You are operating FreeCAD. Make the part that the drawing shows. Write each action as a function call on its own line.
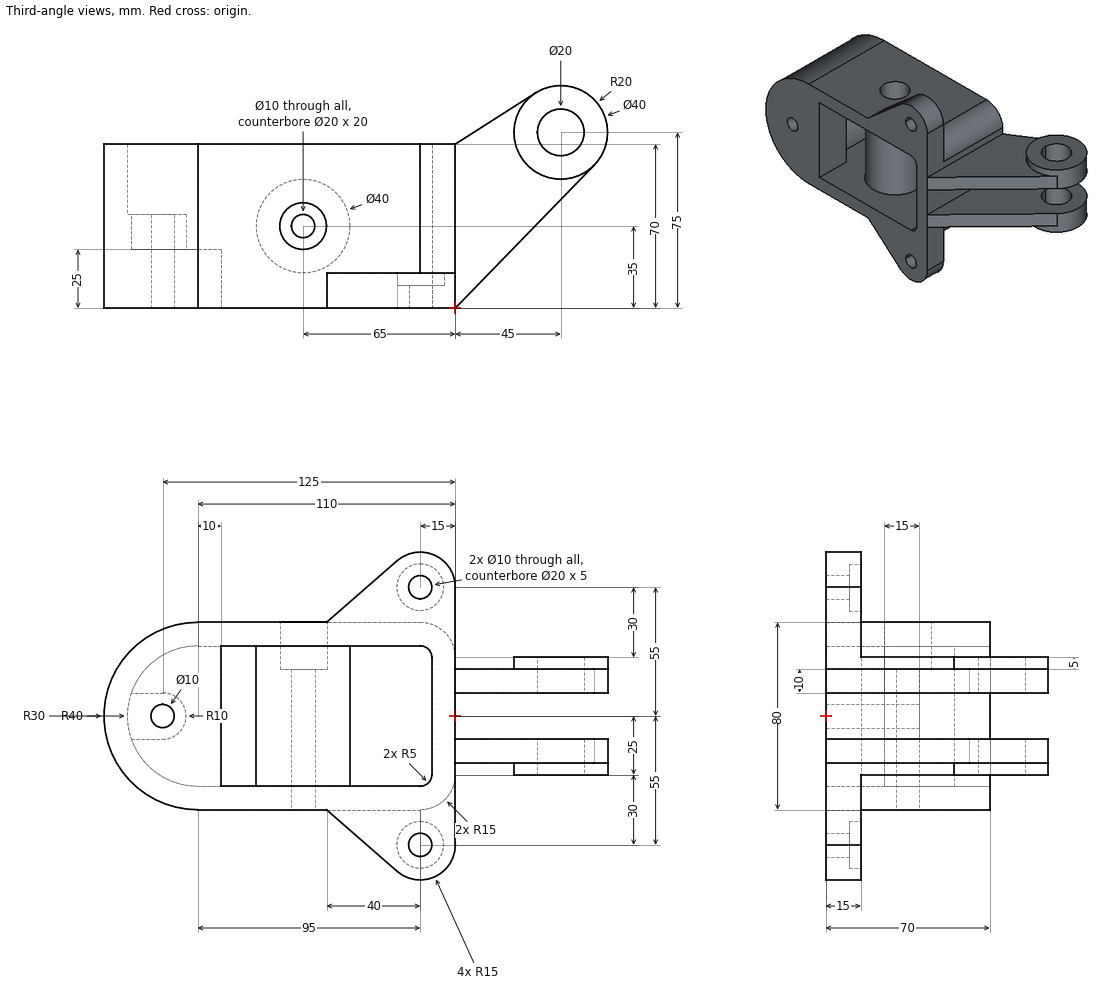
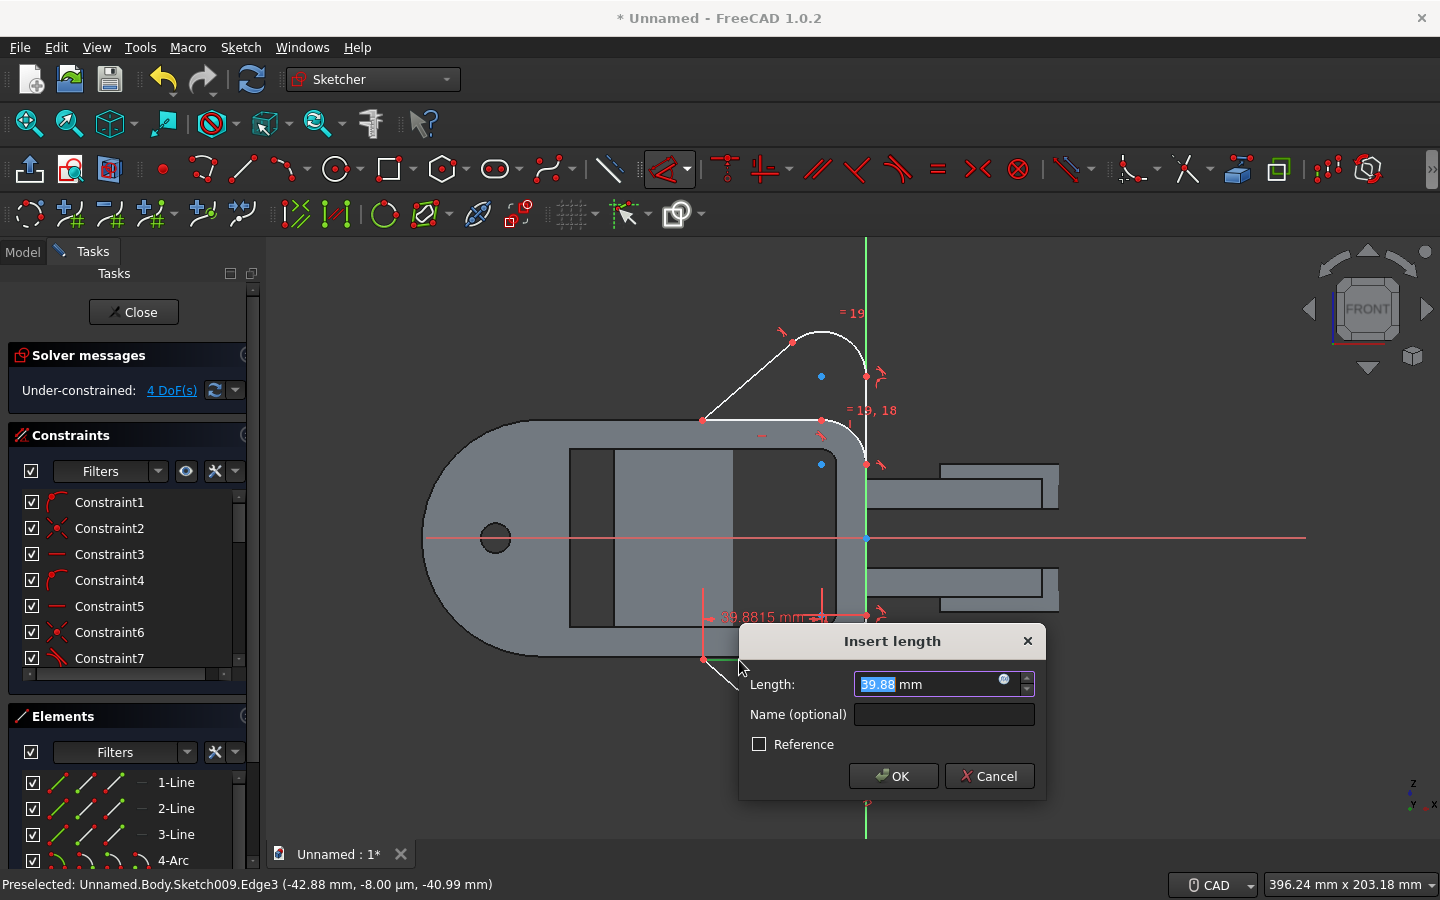
text(40)
key(Return)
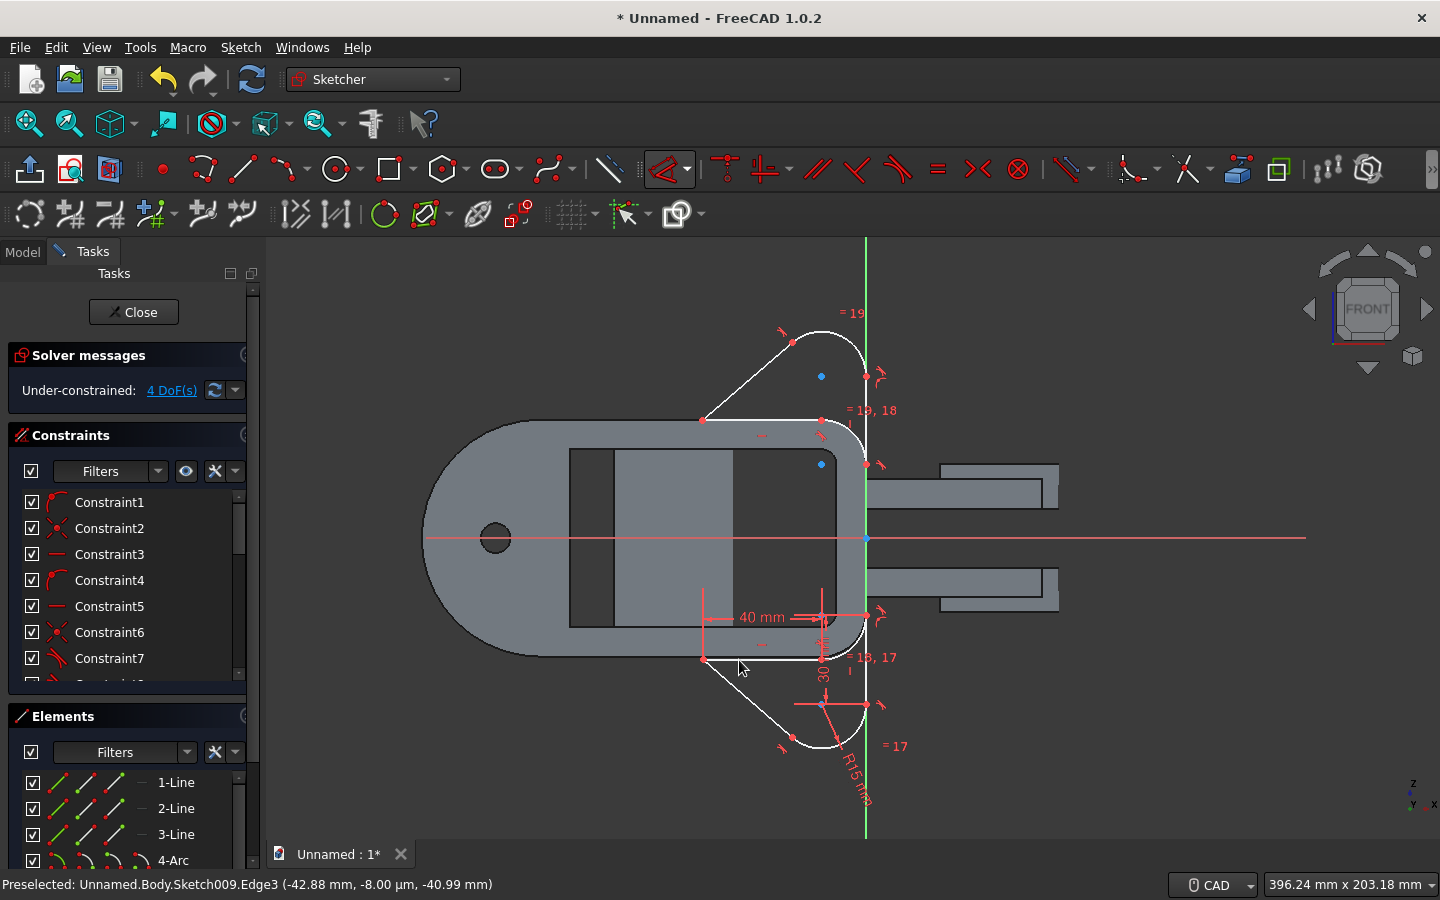
click(866, 429)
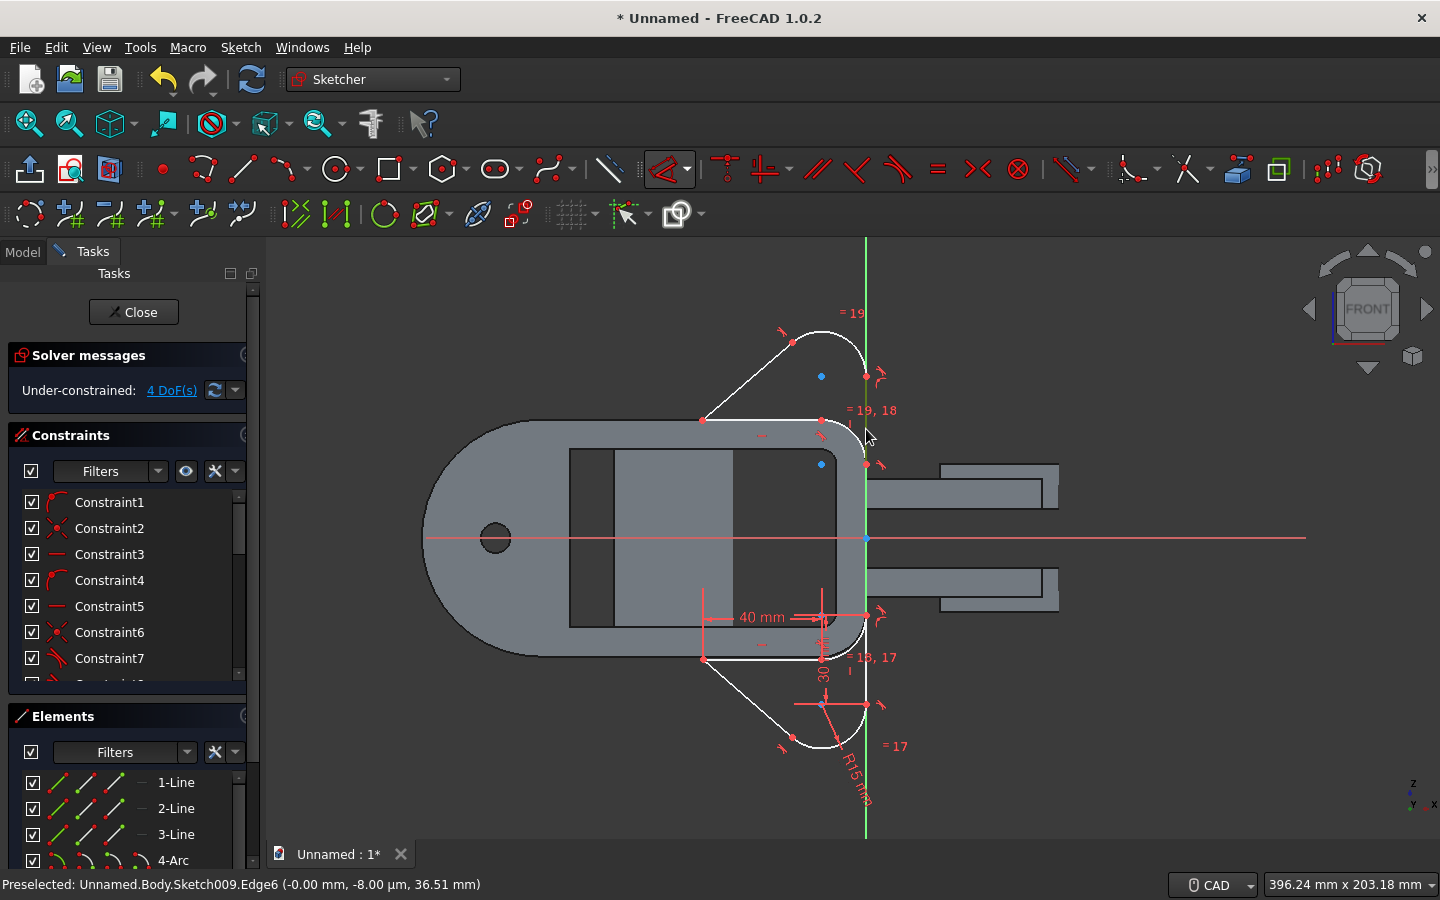
key(i)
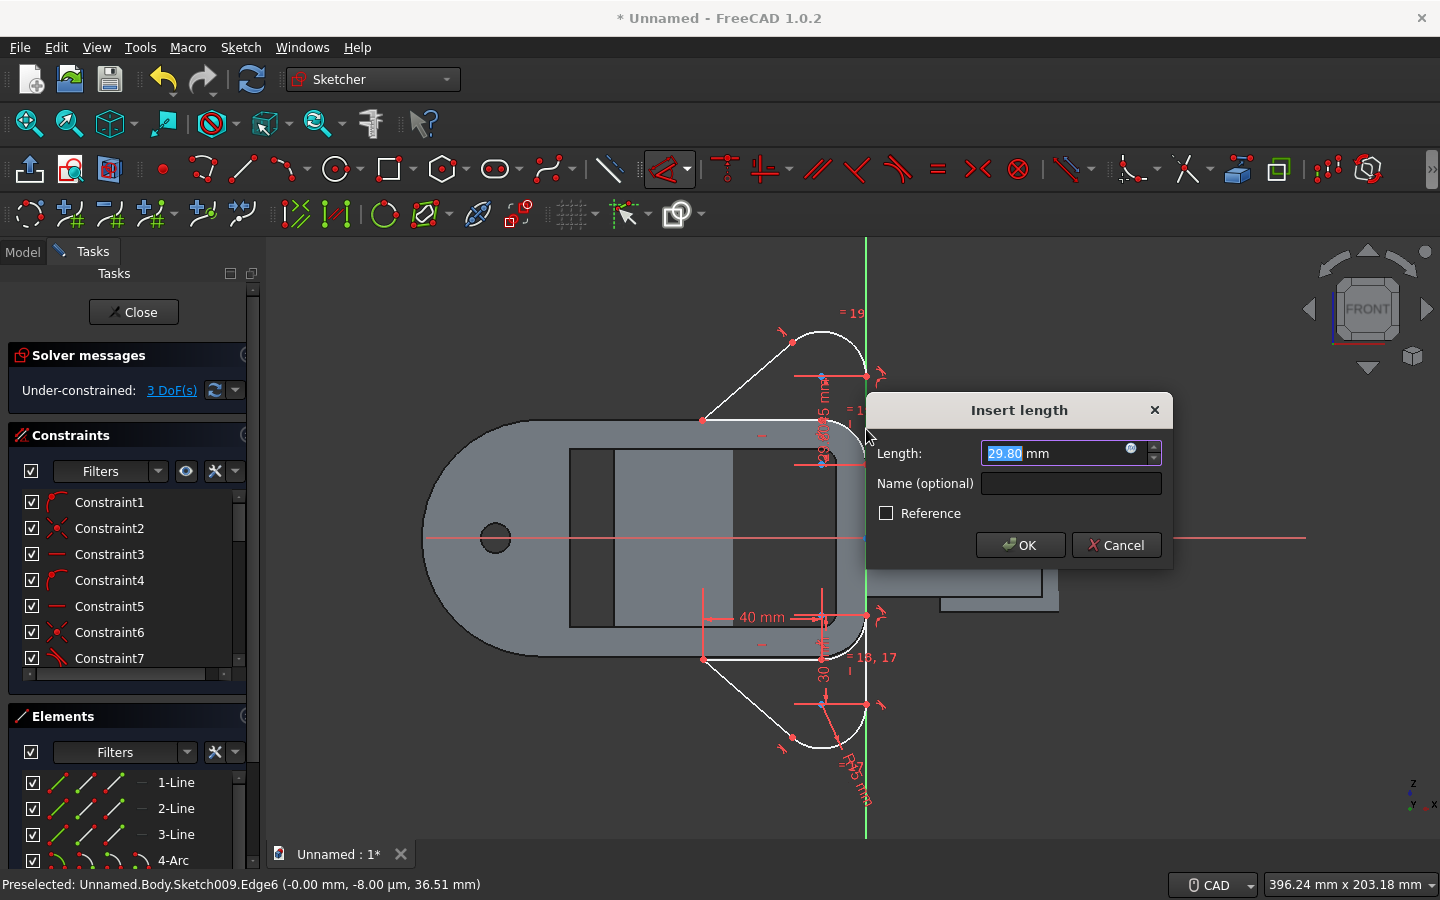
text(30)
key(Return)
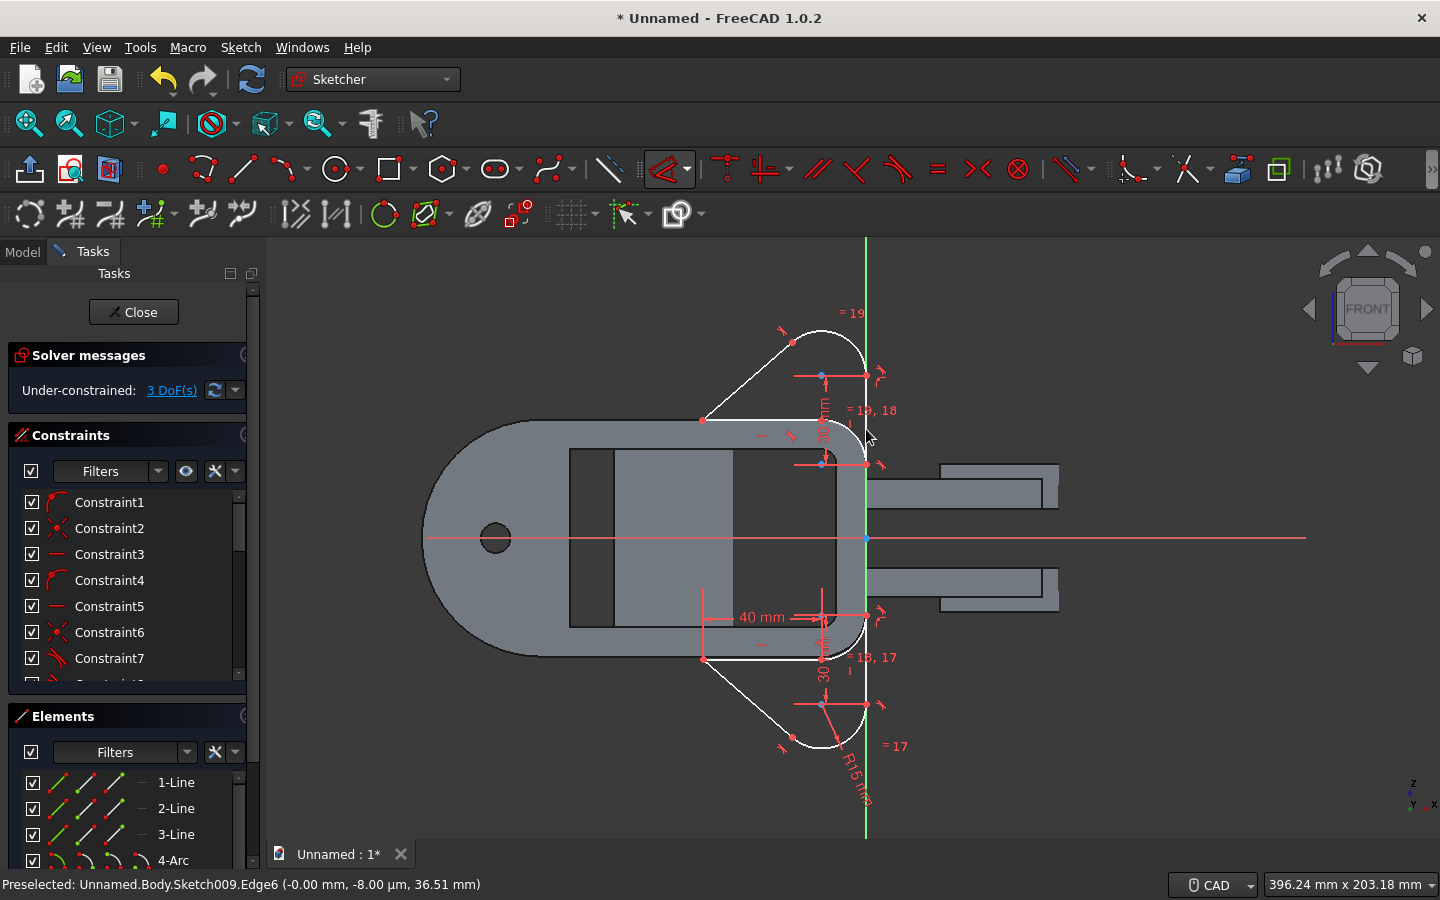
click(786, 420)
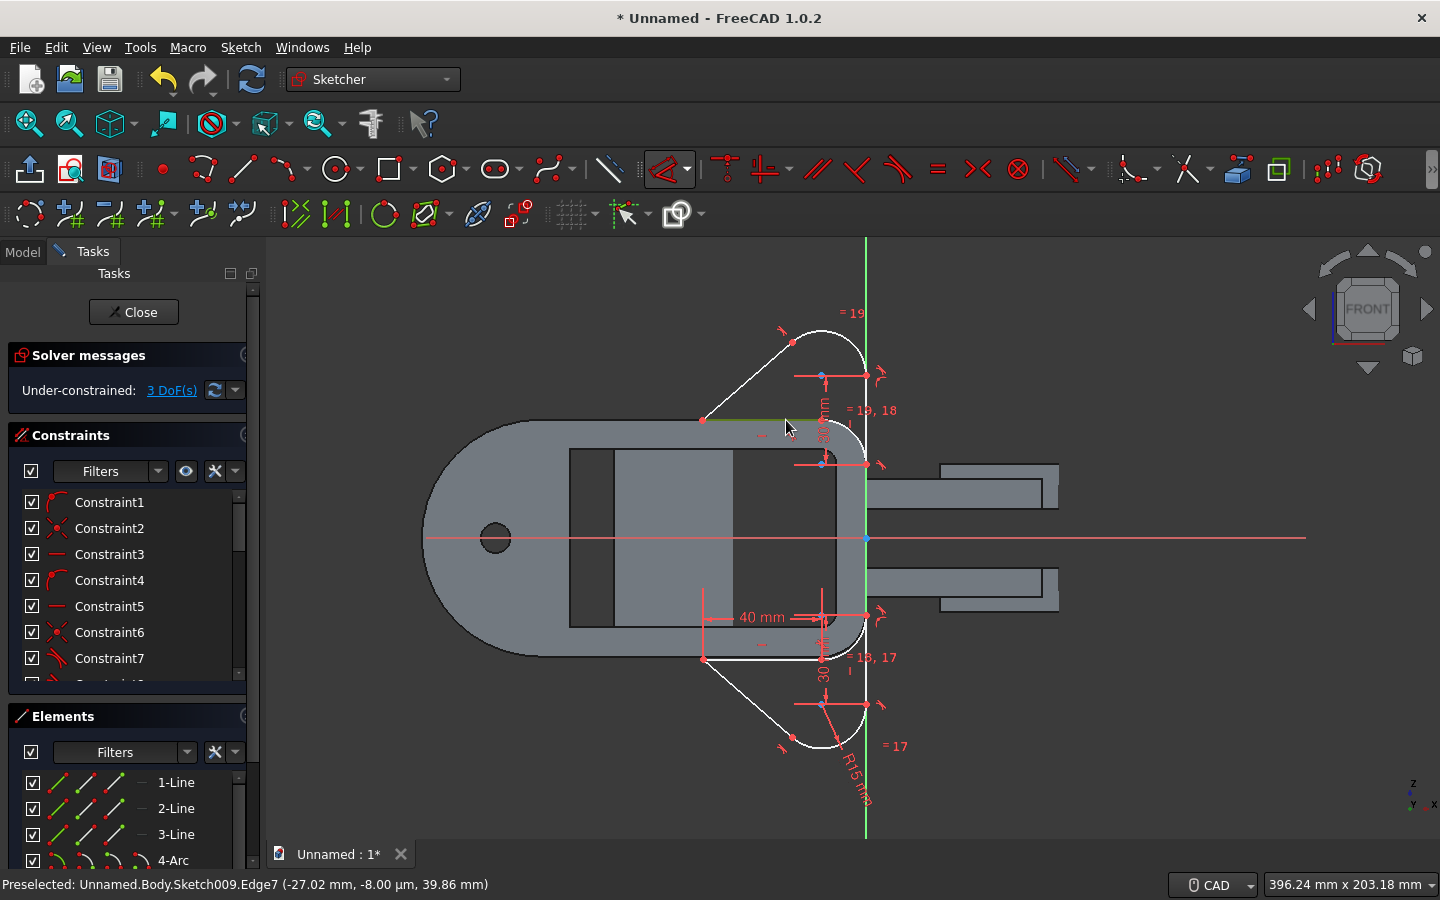
key(l)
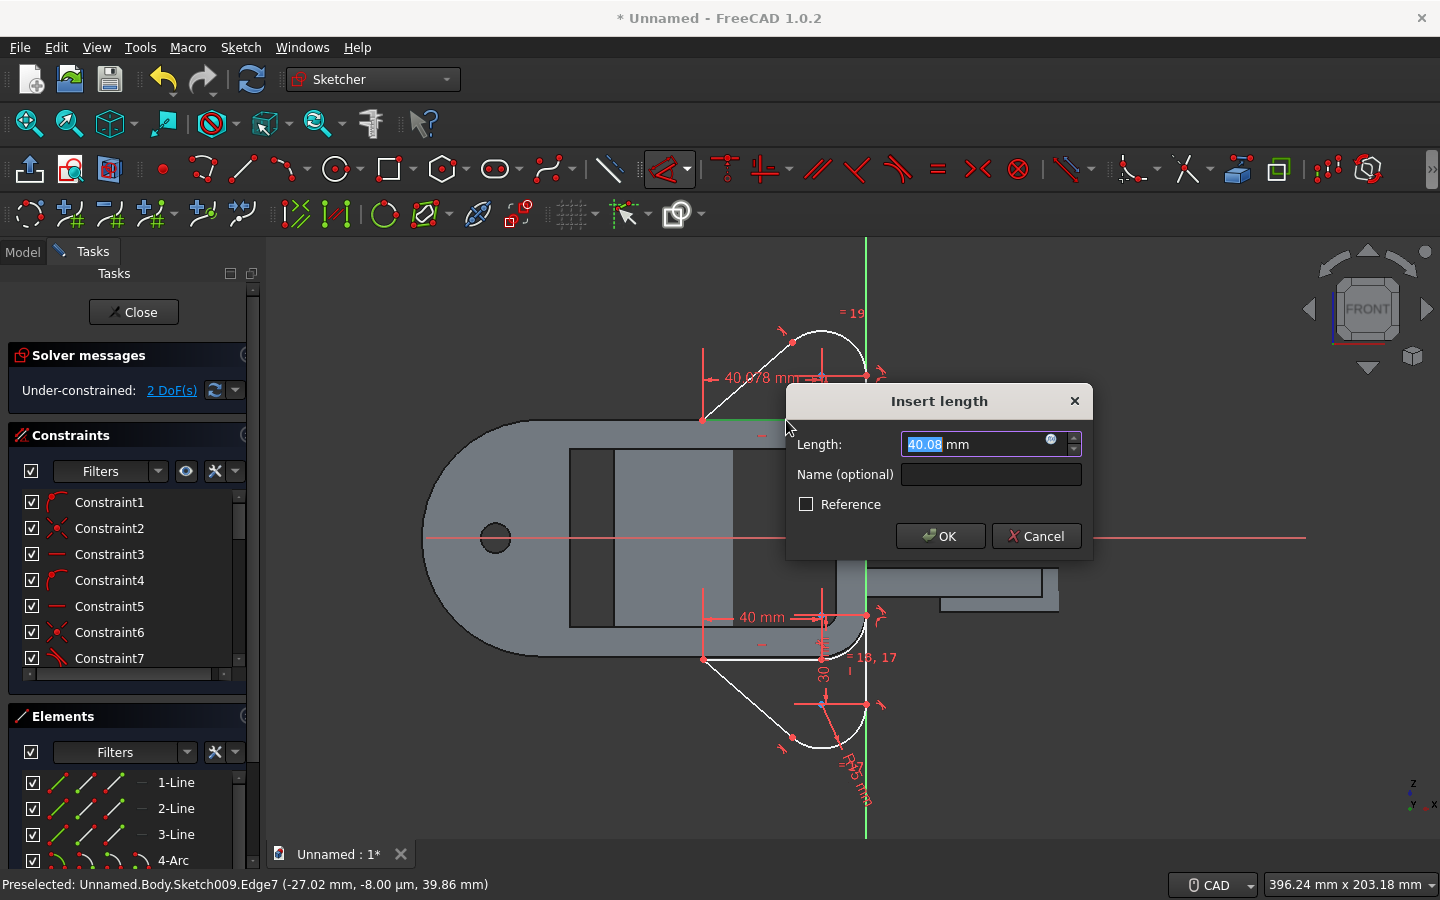
text(40)
key(Return)